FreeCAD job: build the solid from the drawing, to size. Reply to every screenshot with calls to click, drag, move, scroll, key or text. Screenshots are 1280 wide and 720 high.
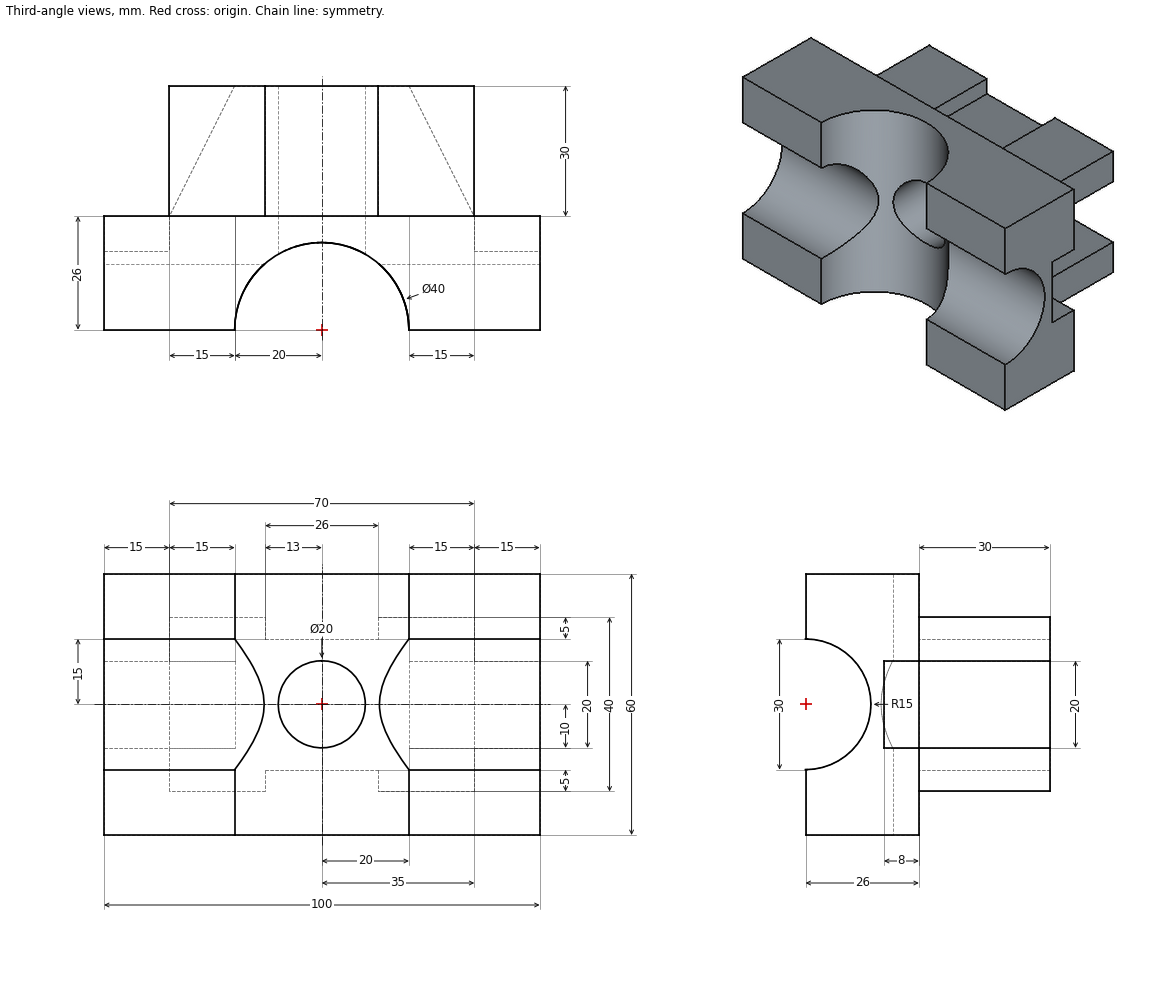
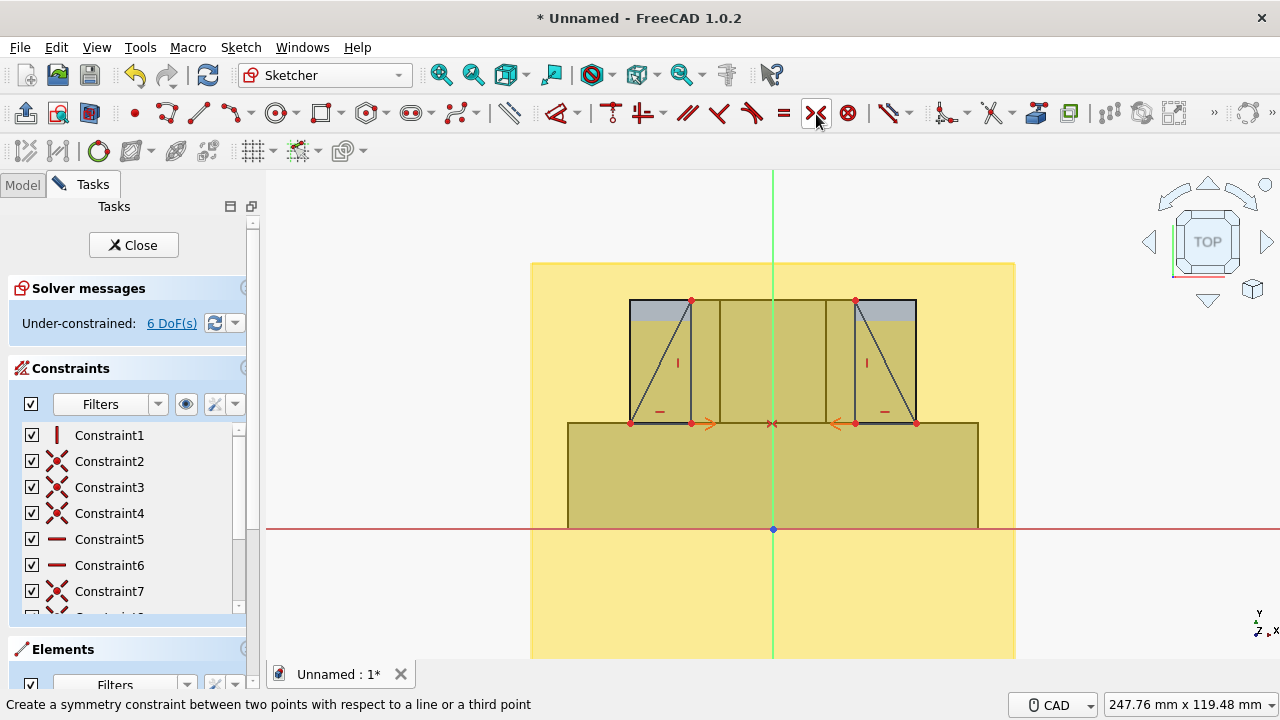
click(691, 387)
click(657, 334)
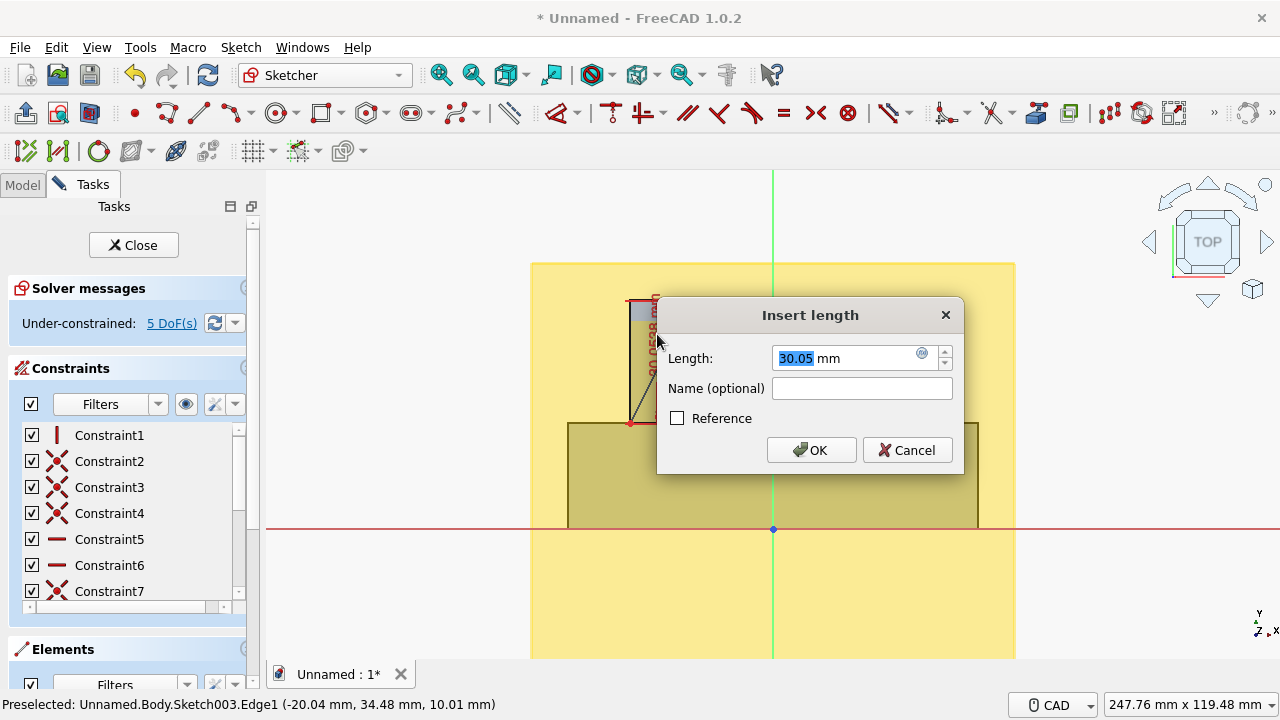
text(30)
key(Return)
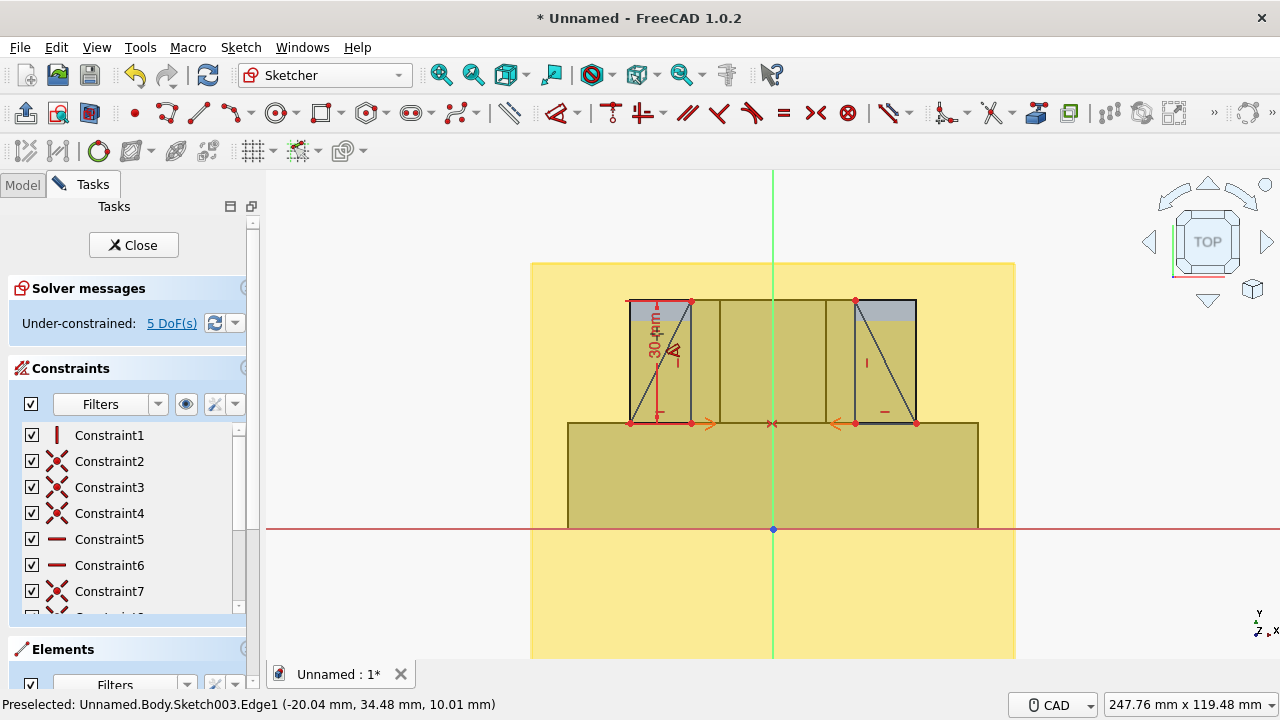
click(648, 424)
click(660, 458)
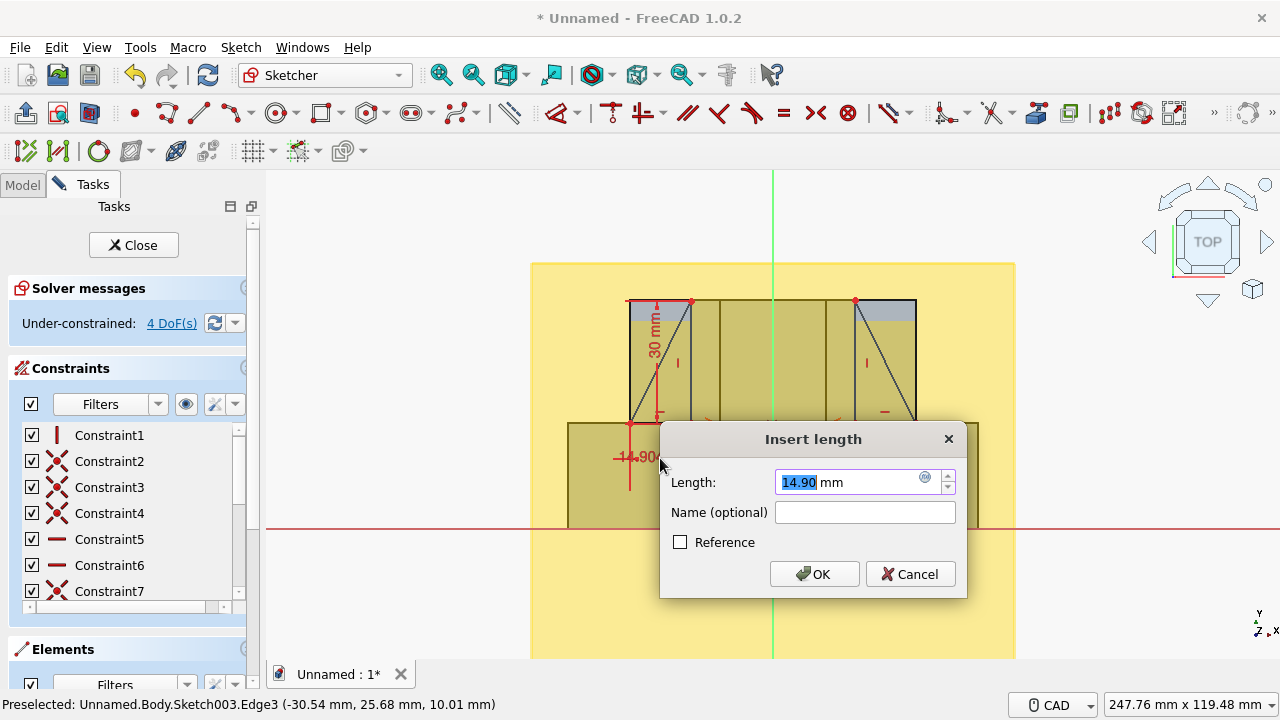
text(15)
key(Return)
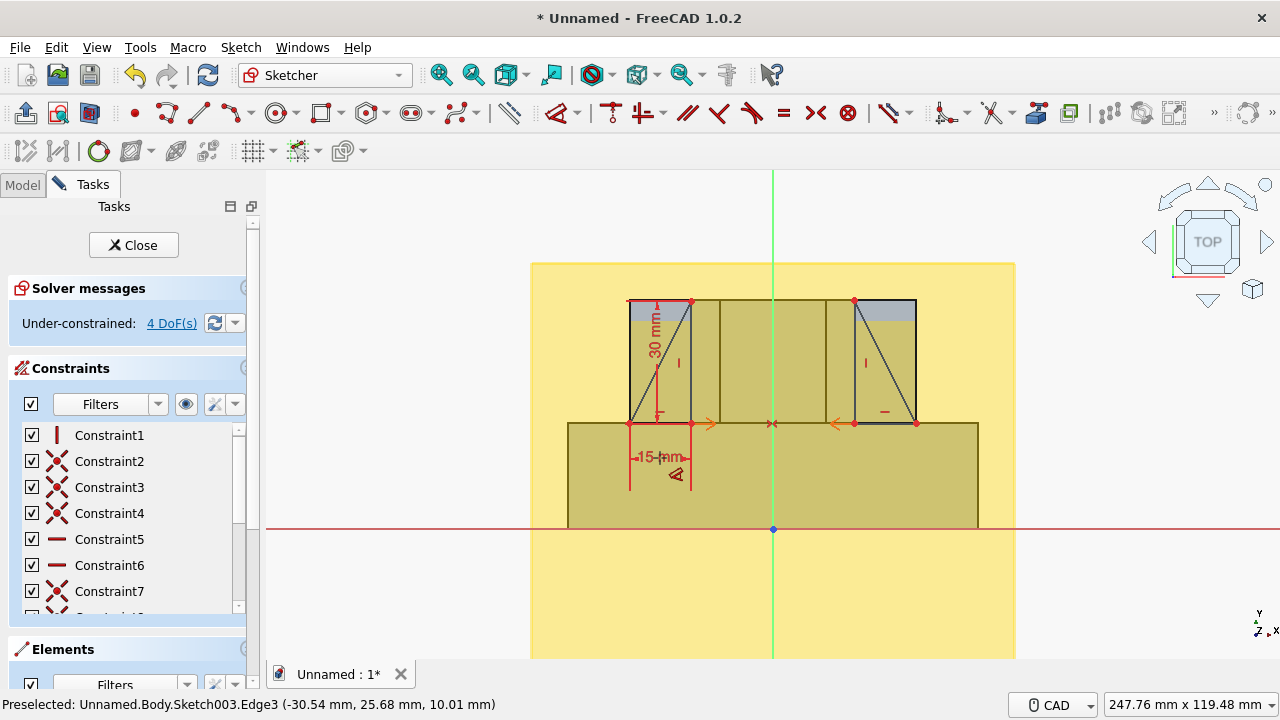
click(873, 424)
click(885, 458)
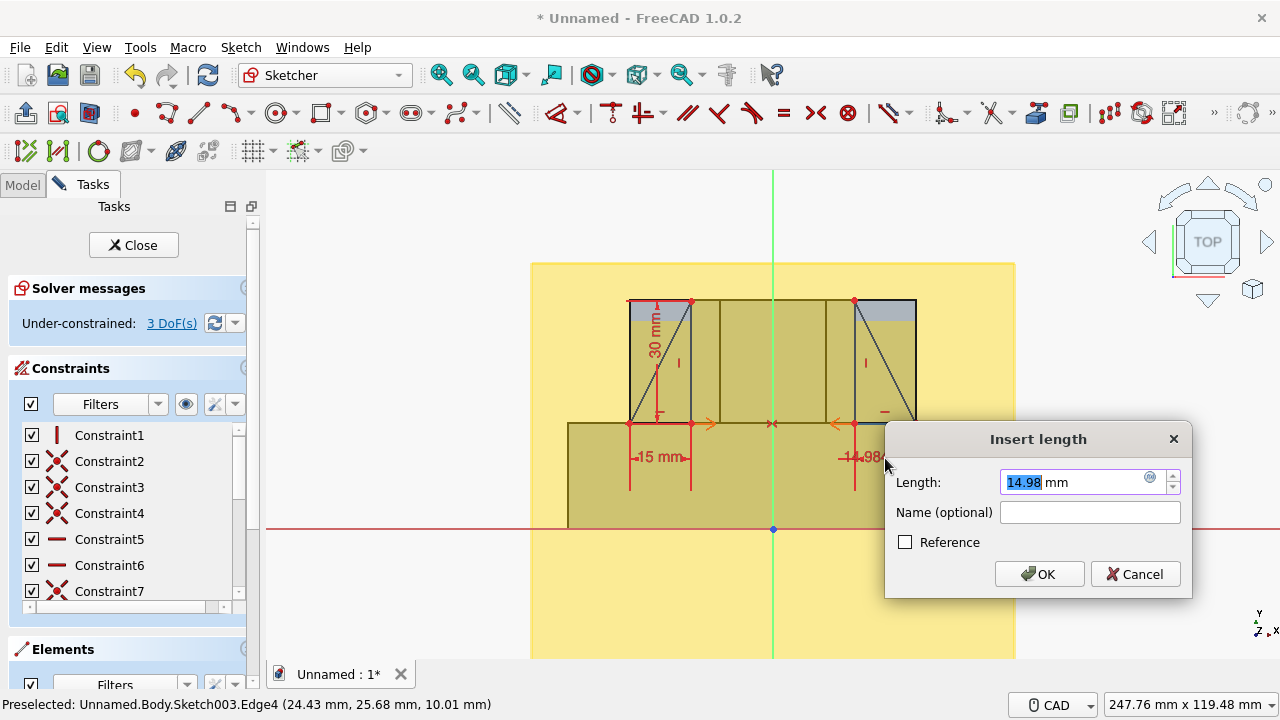
text(15)
key(Return)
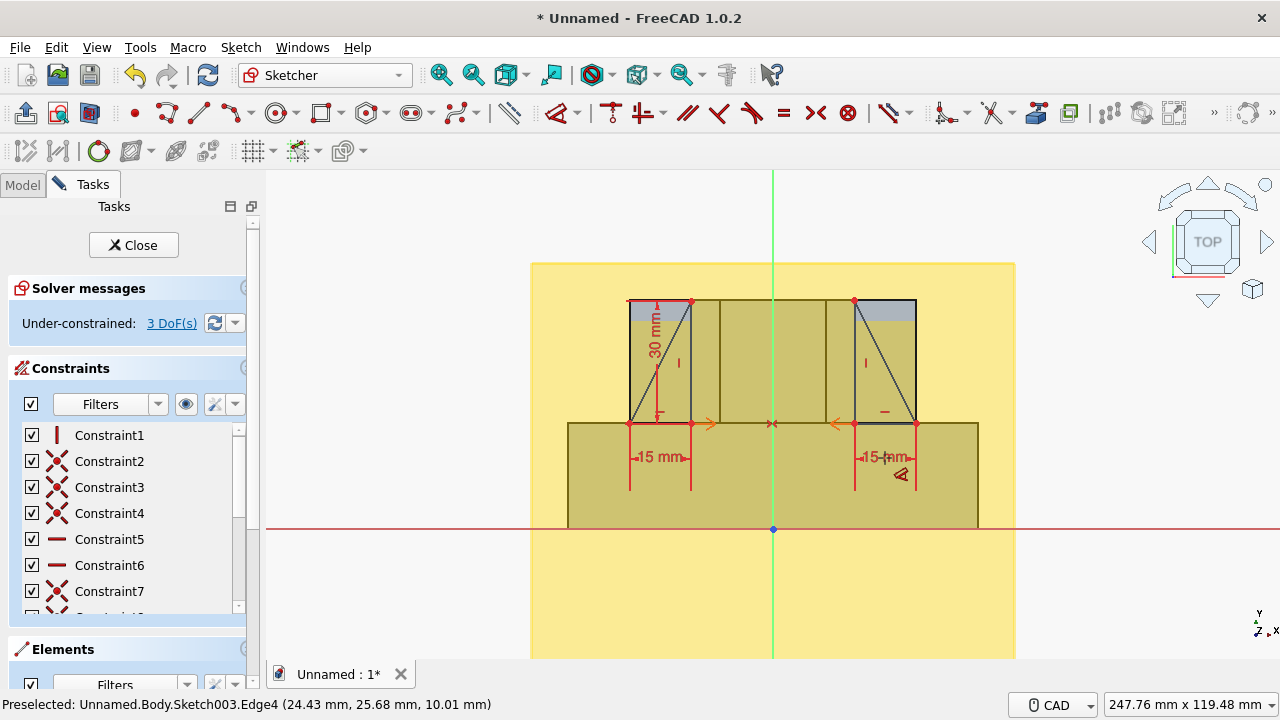
click(855, 338)
click(889, 334)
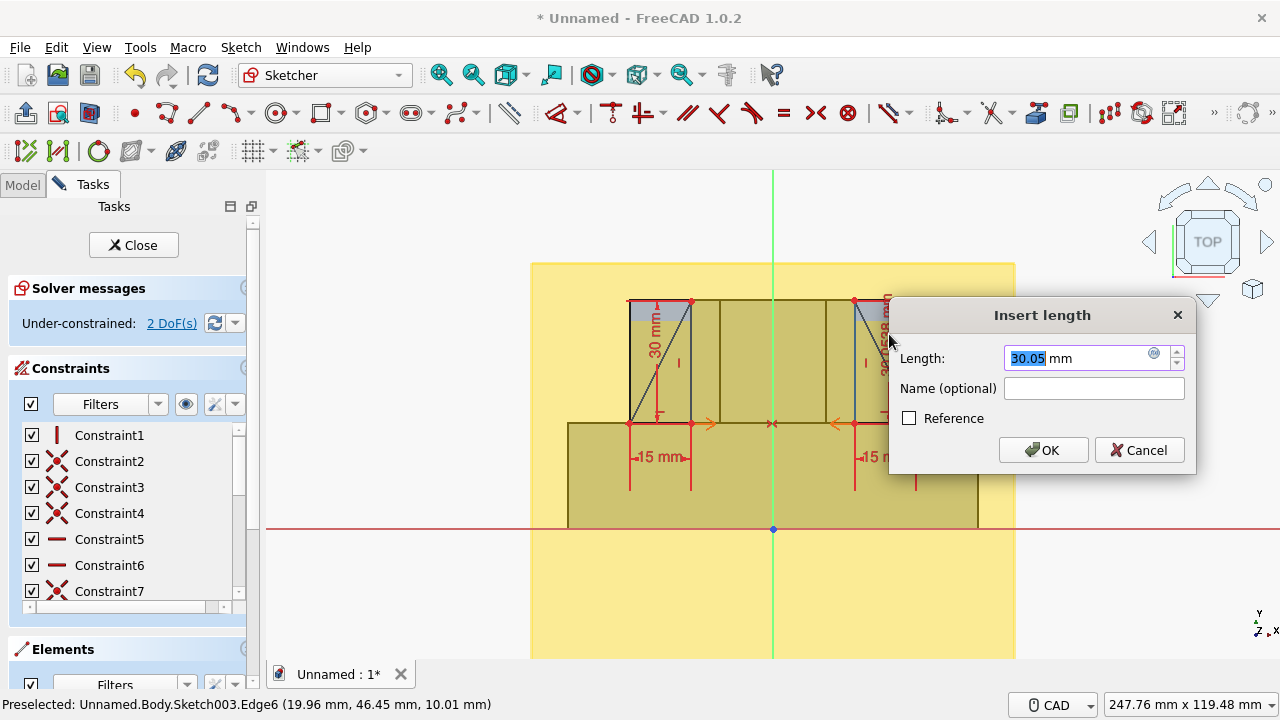
text(30)
key(Return)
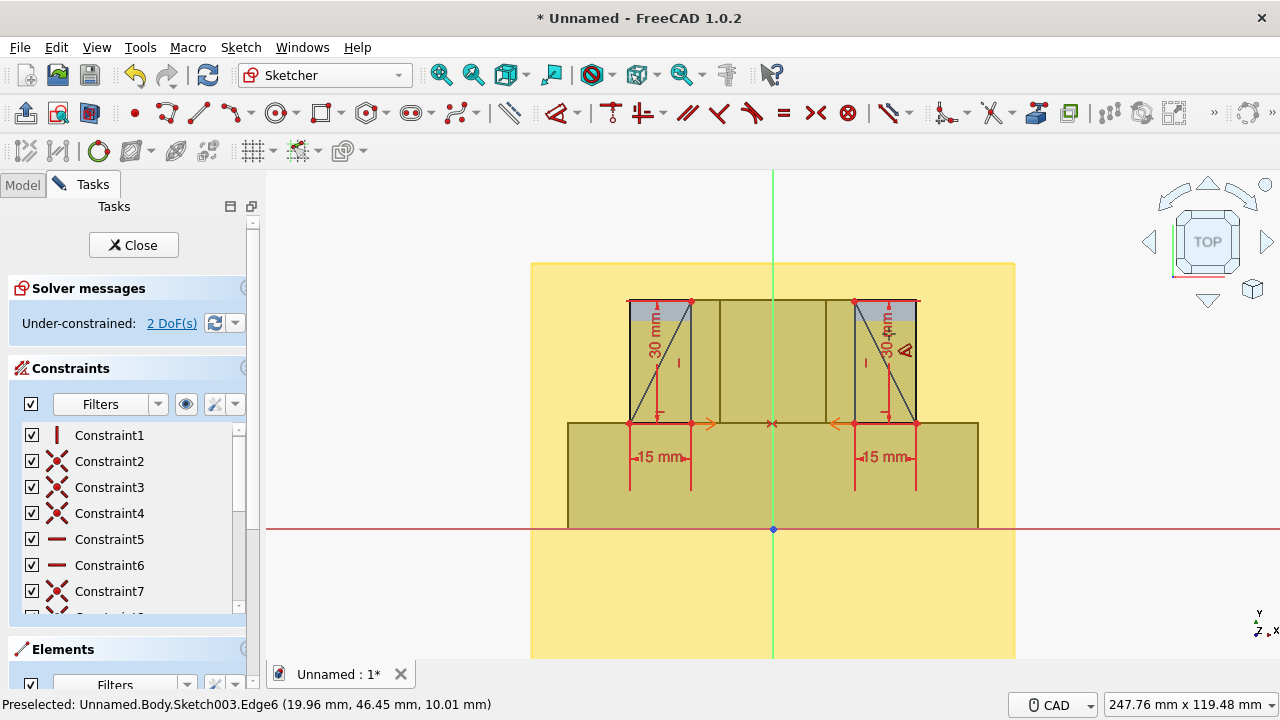
click(691, 424)
click(732, 563)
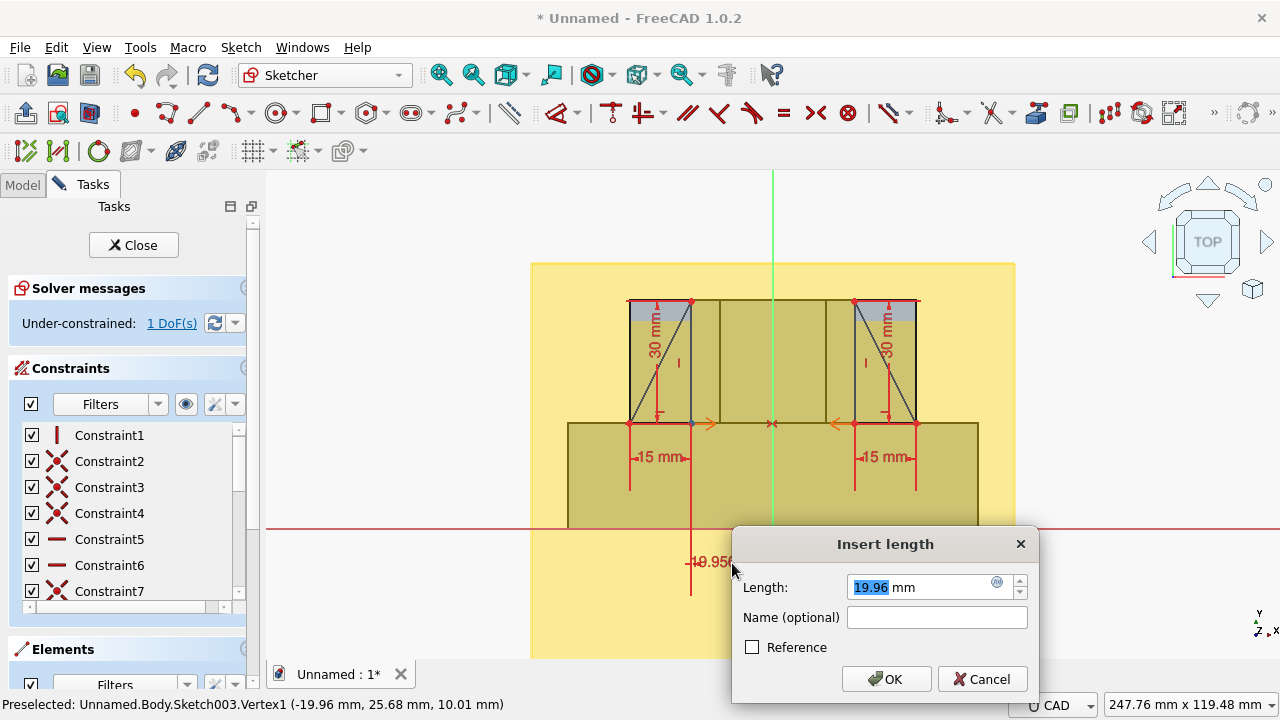
text(20)
key(Return)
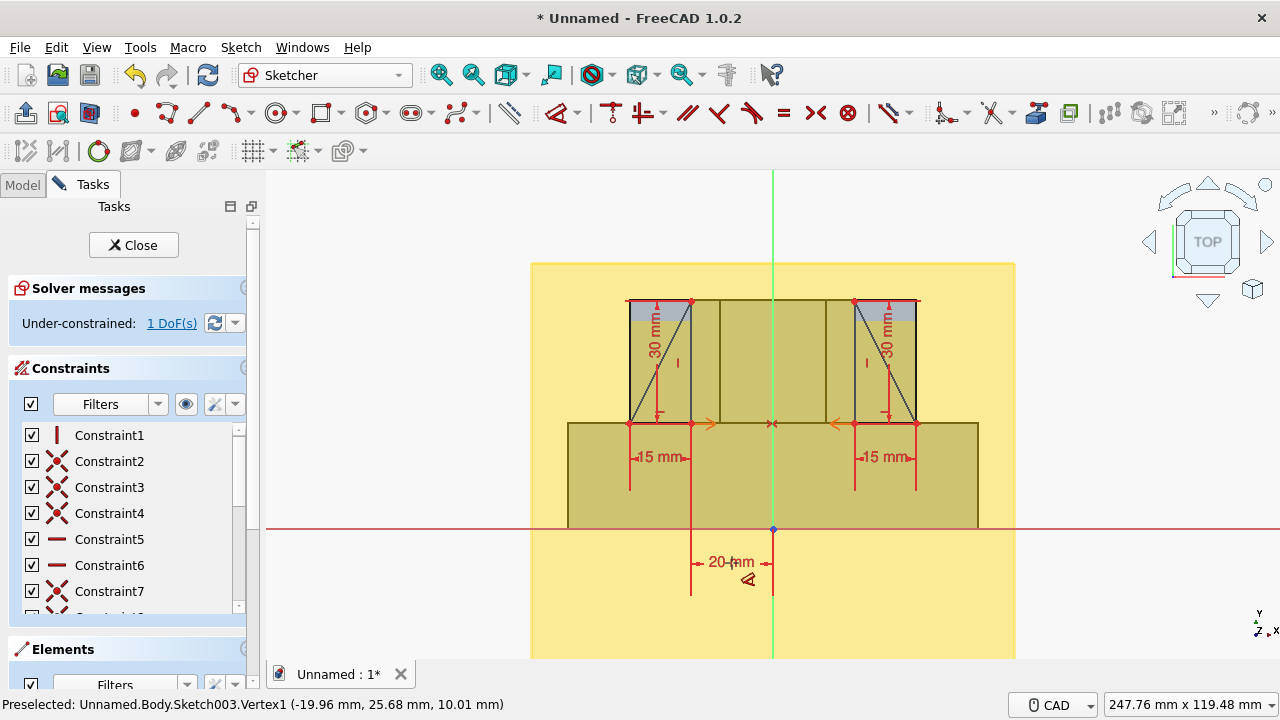
click(691, 424)
click(657, 501)